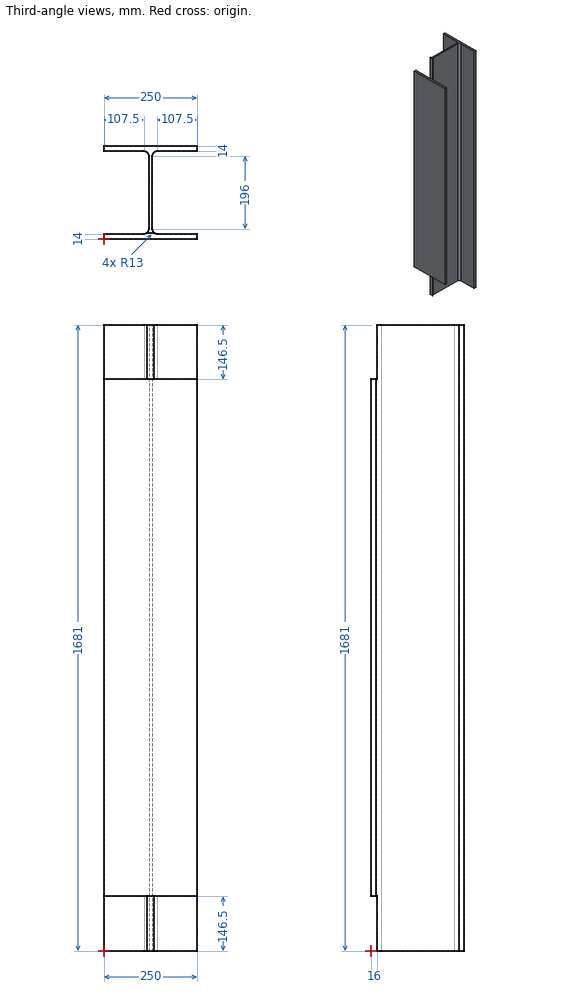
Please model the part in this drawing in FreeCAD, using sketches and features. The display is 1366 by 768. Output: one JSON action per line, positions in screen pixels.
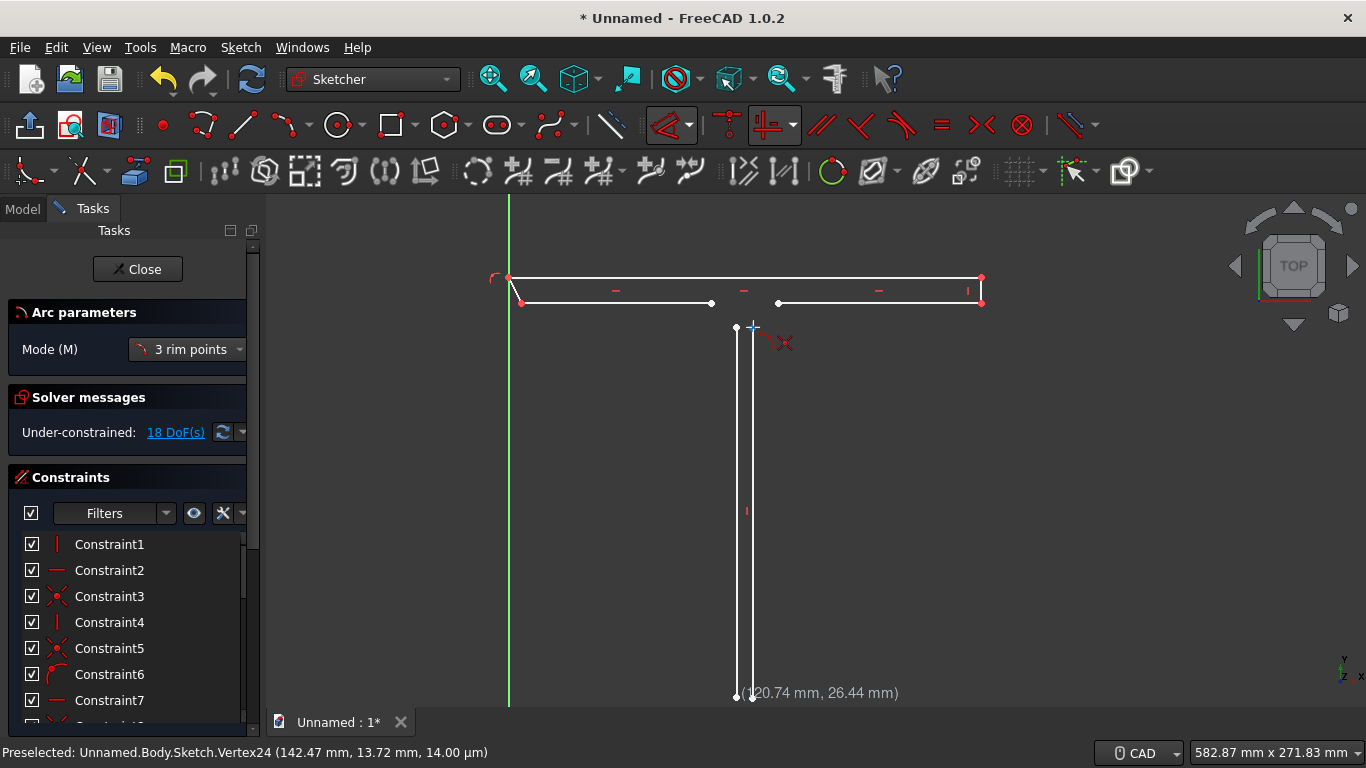
{"action": "left_click", "coordinate": [753, 328]}
{"action": "left_click", "coordinate": [778, 303]}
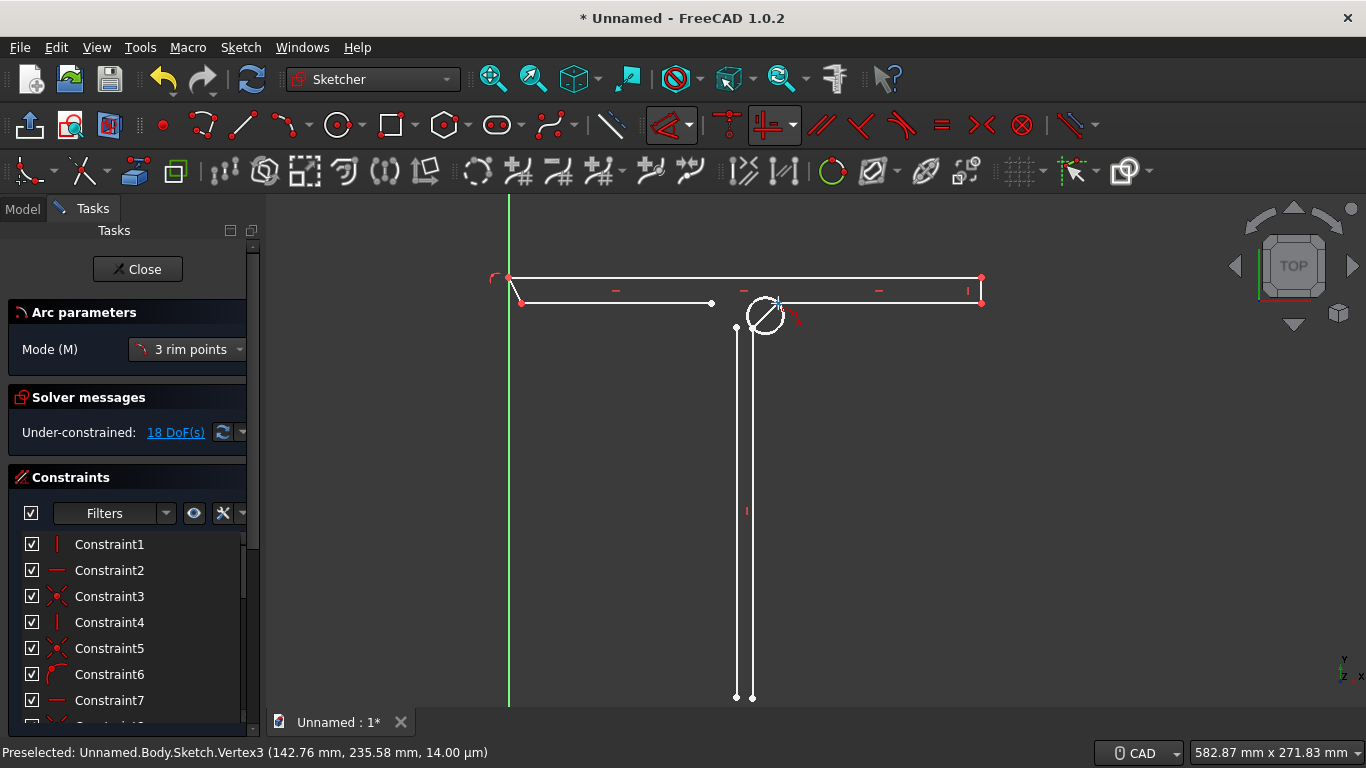
{"action": "scroll", "coordinate": [760, 309], "scroll_direction": "up", "scroll_amount": 4}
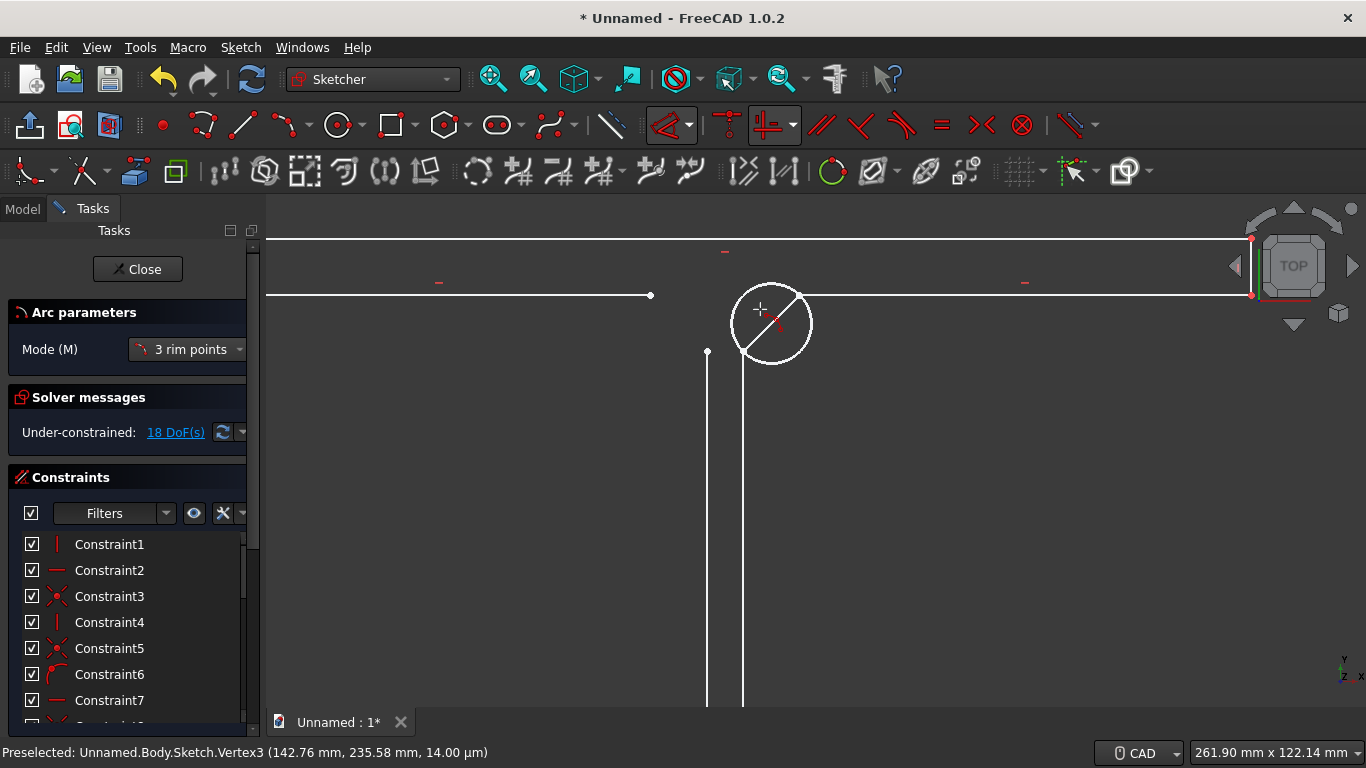
{"action": "left_click", "coordinate": [760, 310]}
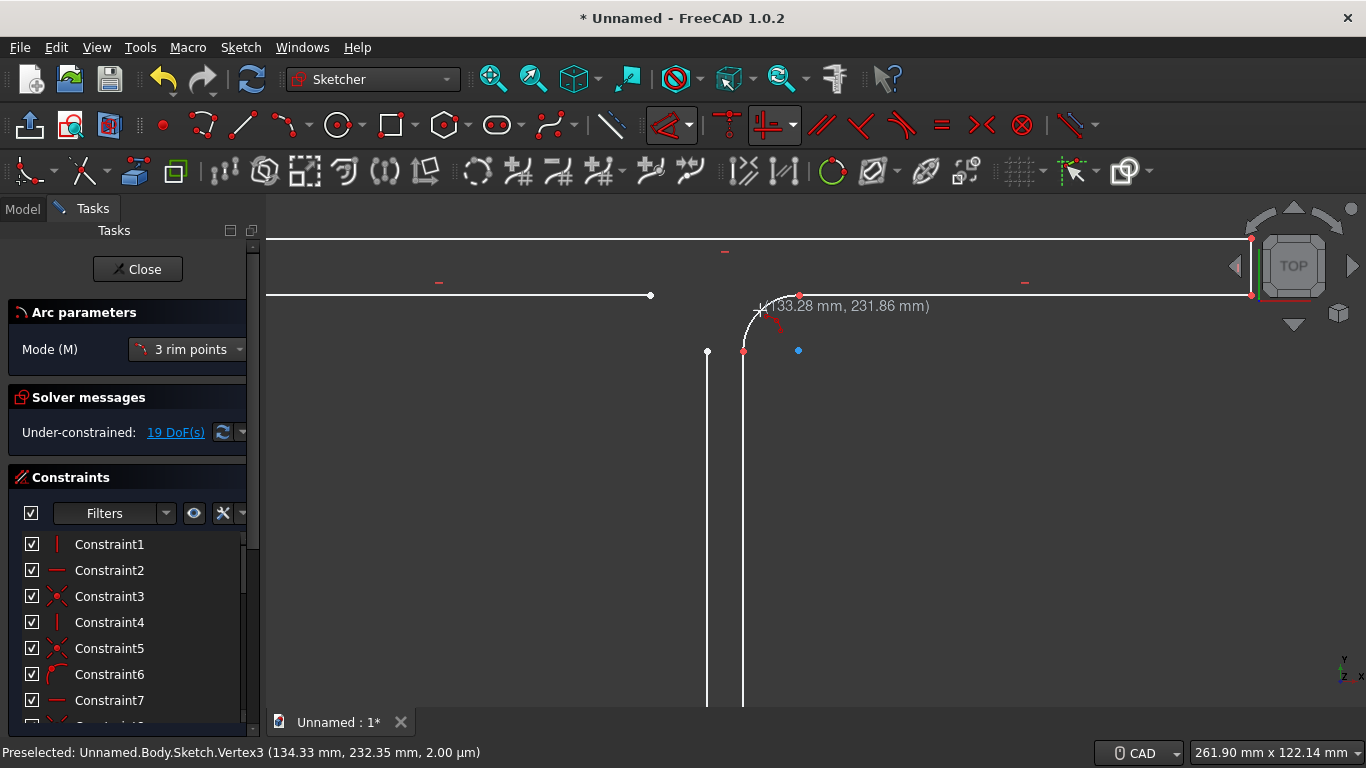
{"action": "left_click", "coordinate": [650, 295]}
{"action": "left_click", "coordinate": [707, 351]}
{"action": "left_click", "coordinate": [690, 310]}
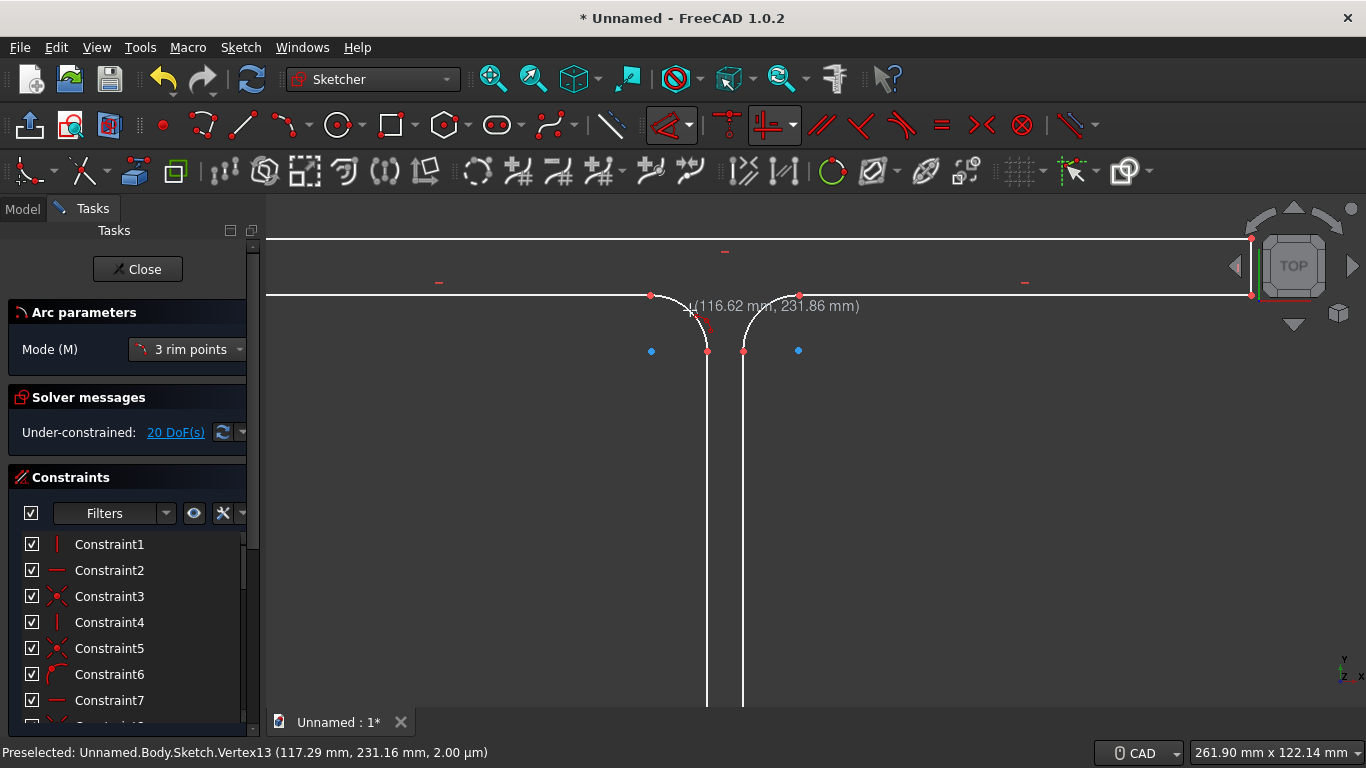
{"action": "scroll", "coordinate": [757, 317], "scroll_direction": "down", "scroll_amount": 6}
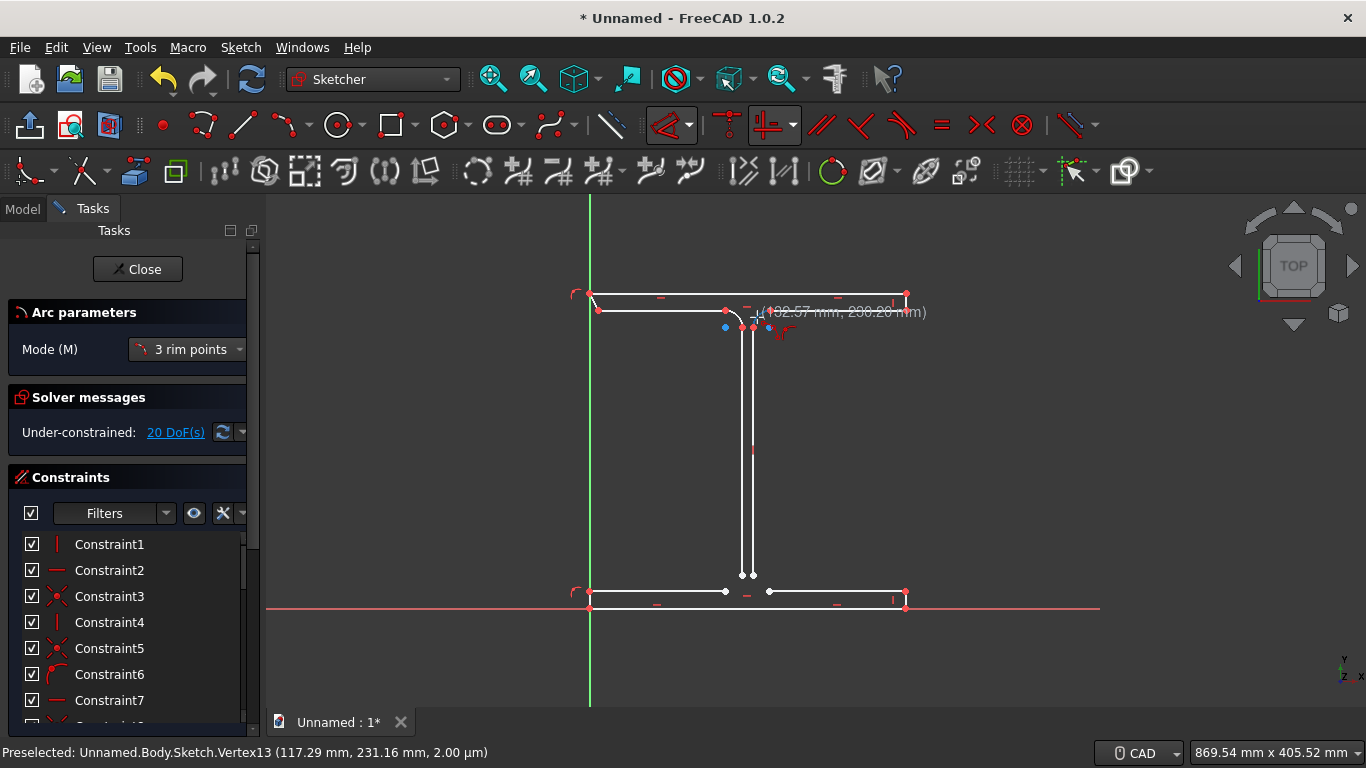
{"action": "scroll", "coordinate": [742, 575], "scroll_direction": "up", "scroll_amount": 2}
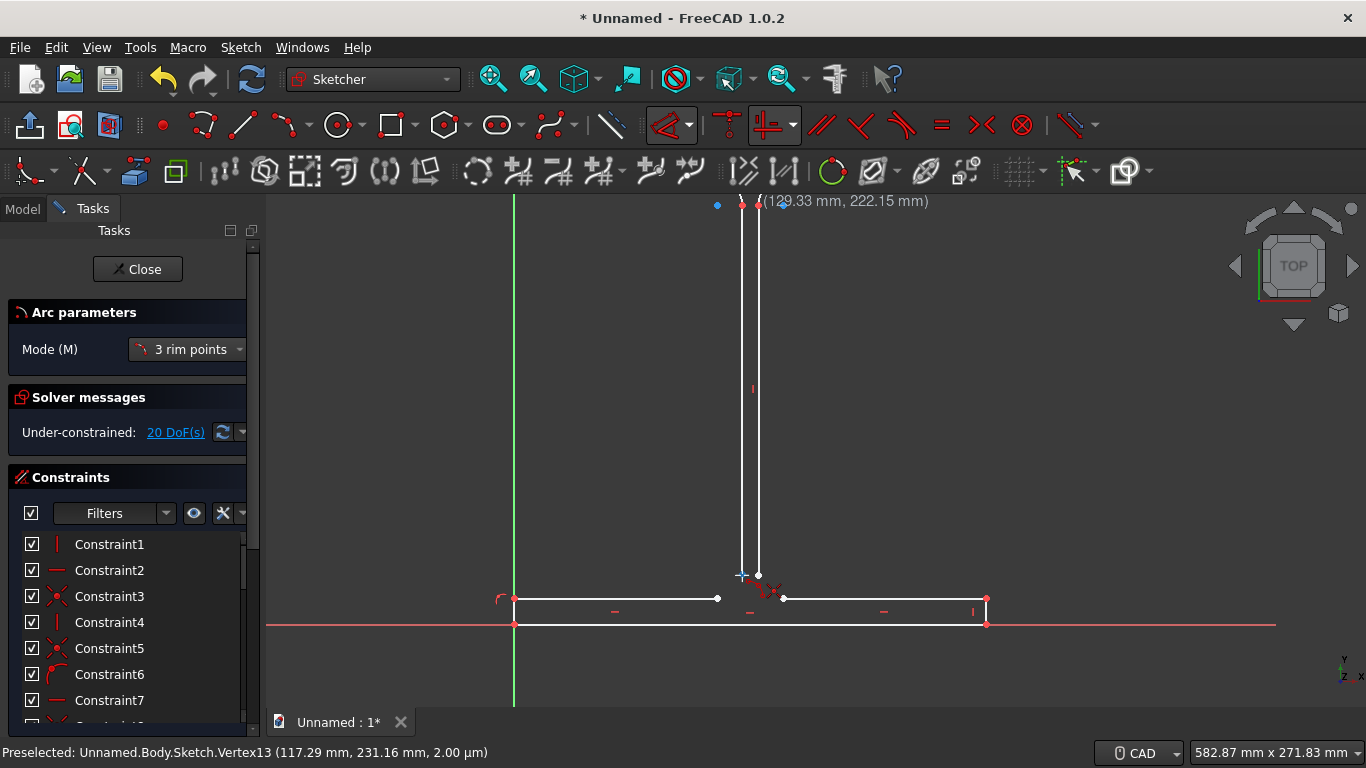
{"action": "left_click", "coordinate": [742, 575]}
{"action": "left_click", "coordinate": [717, 599]}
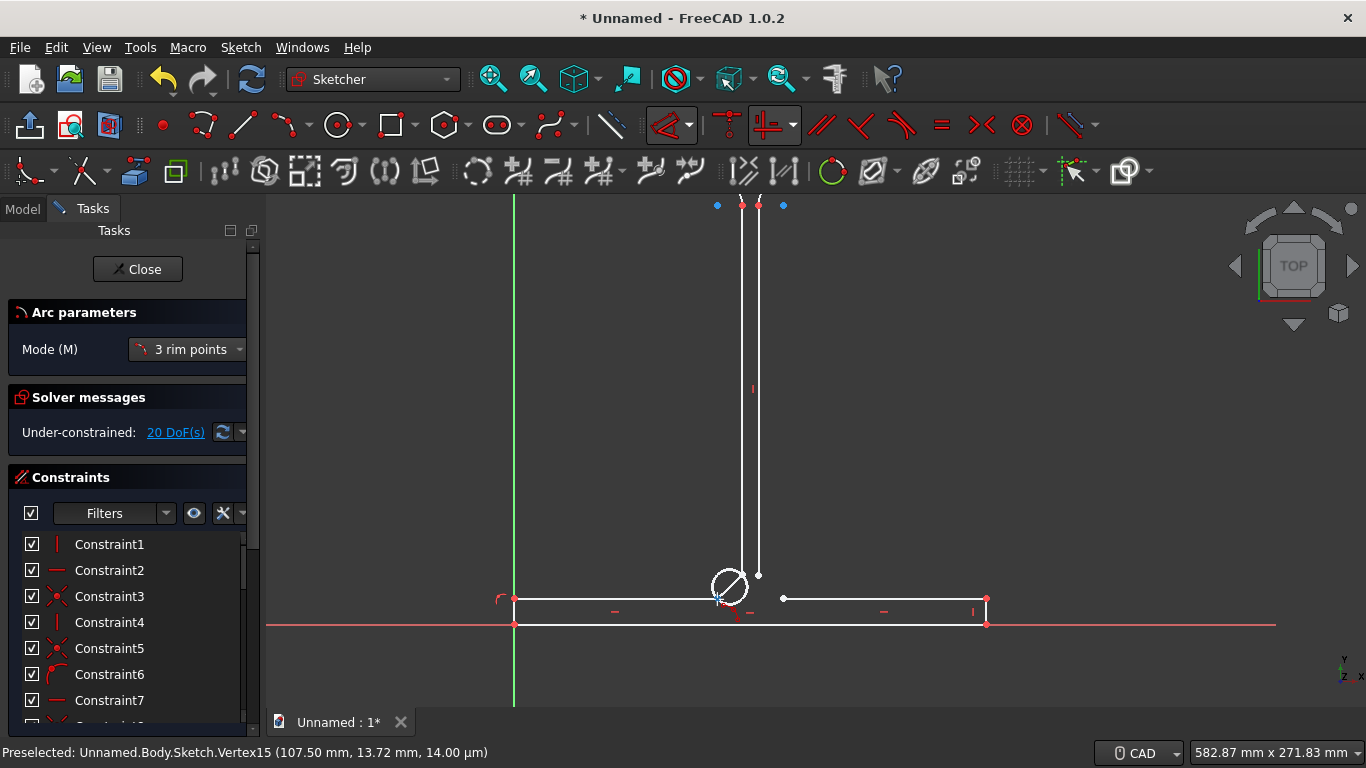
{"action": "scroll", "coordinate": [735, 591], "scroll_direction": "up", "scroll_amount": 4}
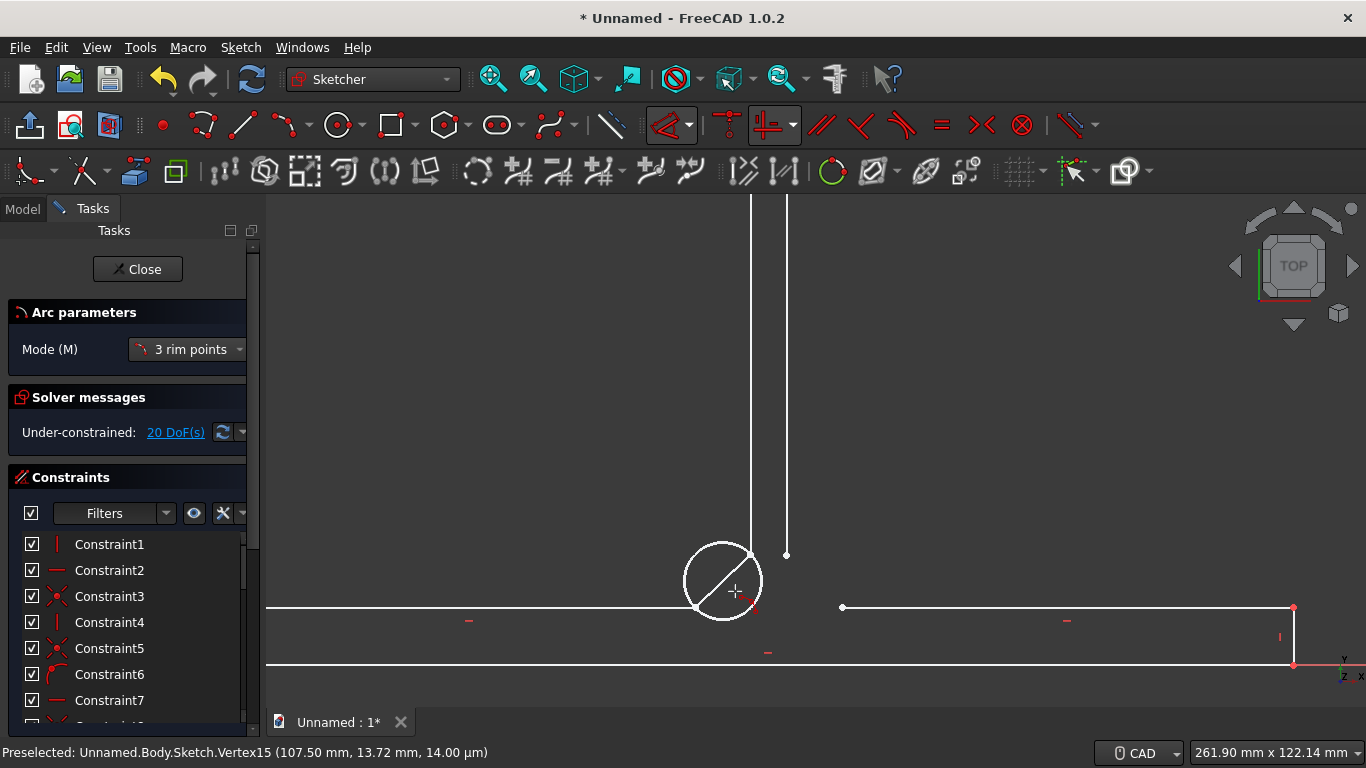
{"action": "left_click", "coordinate": [734, 591]}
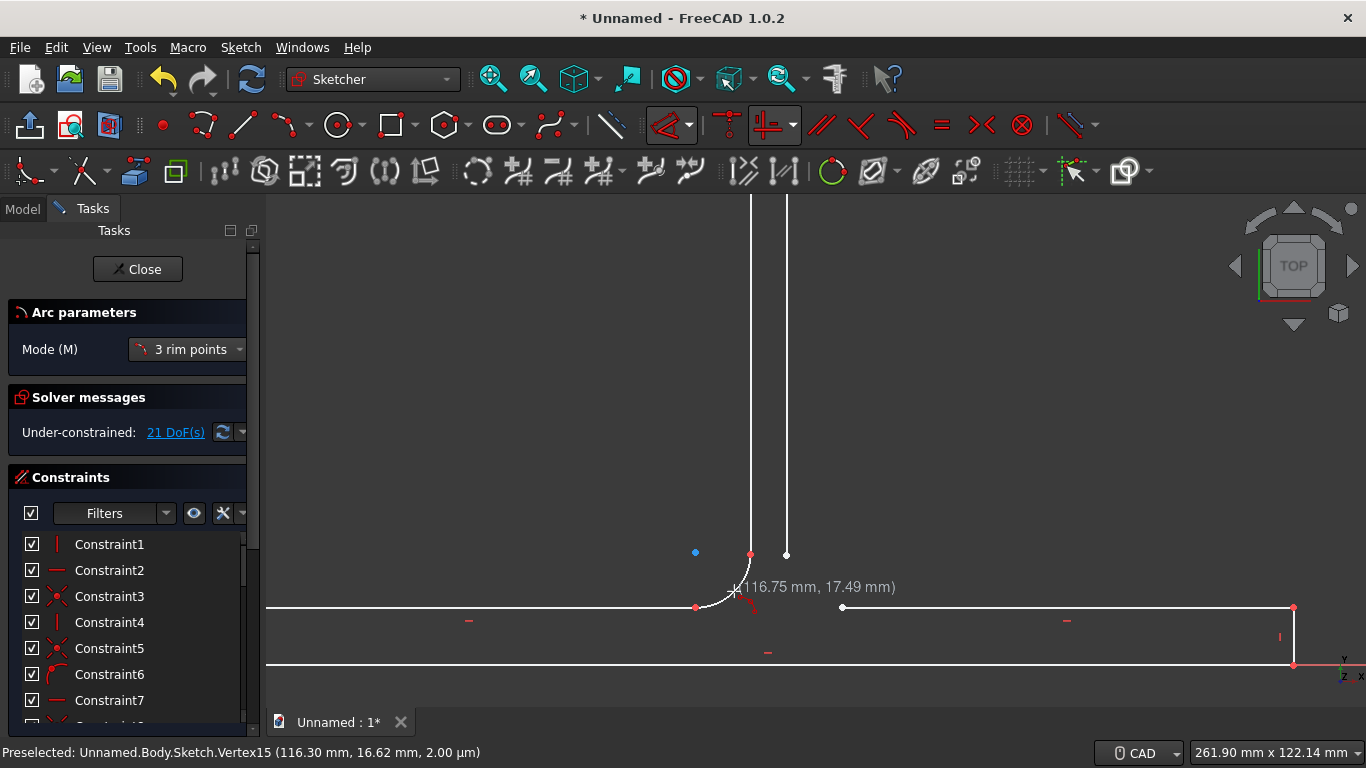
{"action": "left_click", "coordinate": [842, 608]}
{"action": "left_click", "coordinate": [787, 556]}
{"action": "left_click", "coordinate": [804, 591]}
{"action": "key", "text": "Escape"}